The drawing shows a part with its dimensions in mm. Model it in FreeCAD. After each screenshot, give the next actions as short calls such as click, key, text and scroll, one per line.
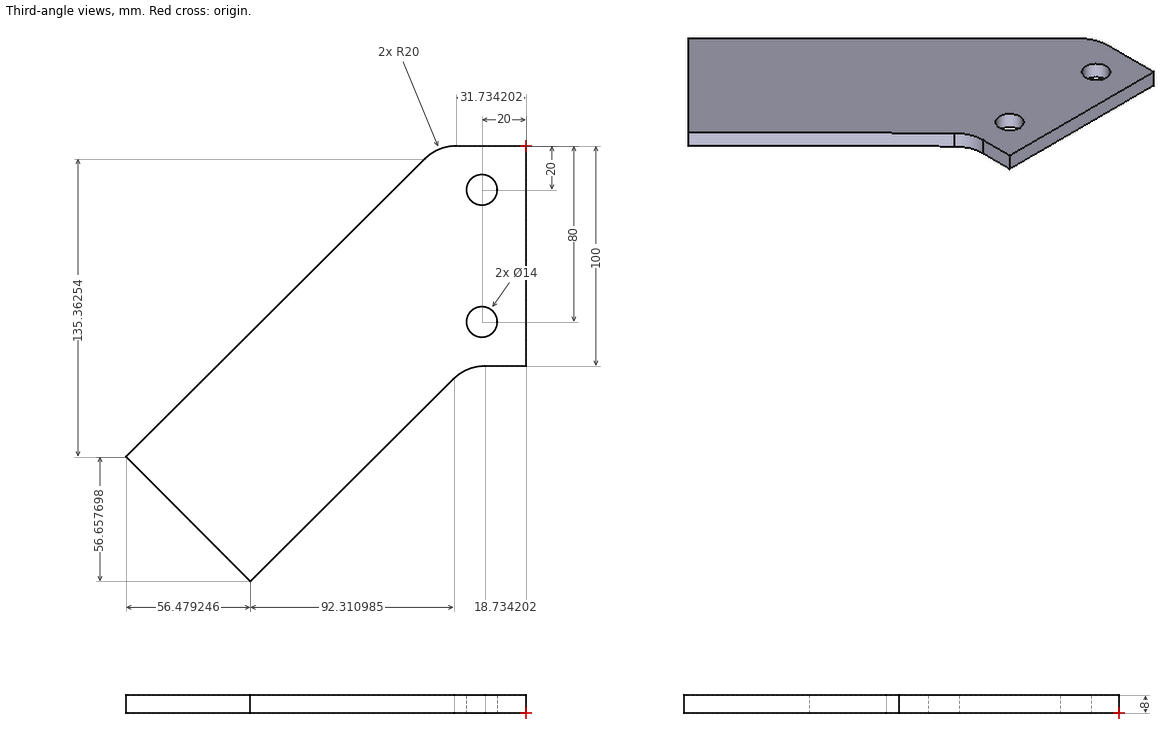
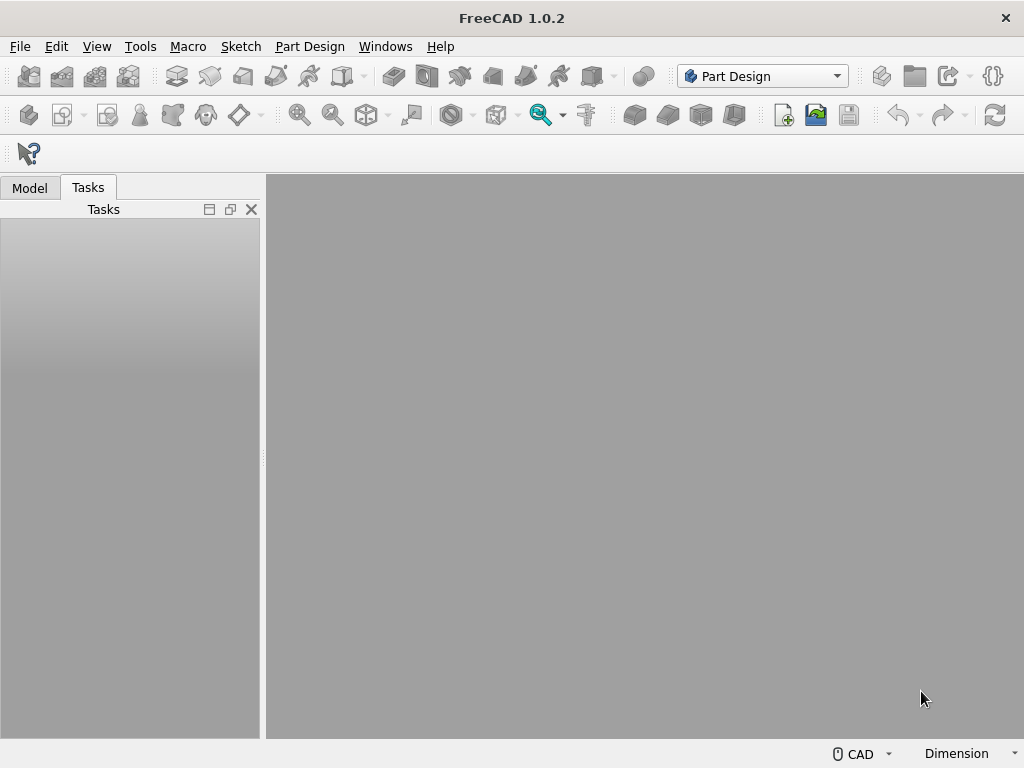
click(783, 116)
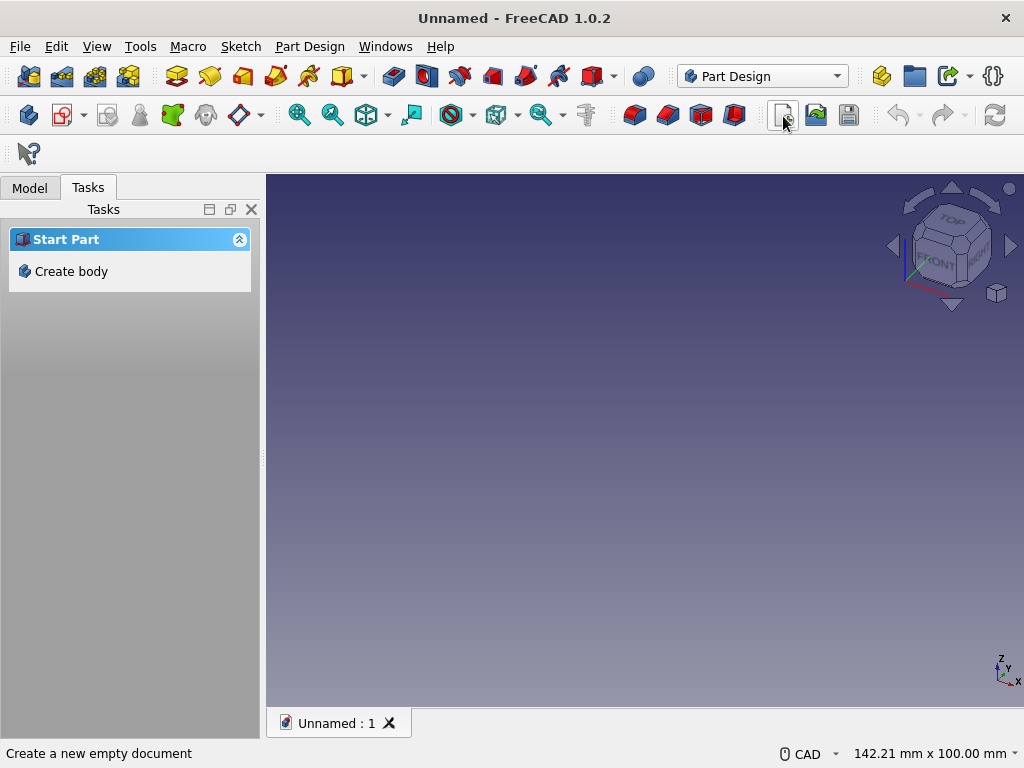
click(62, 116)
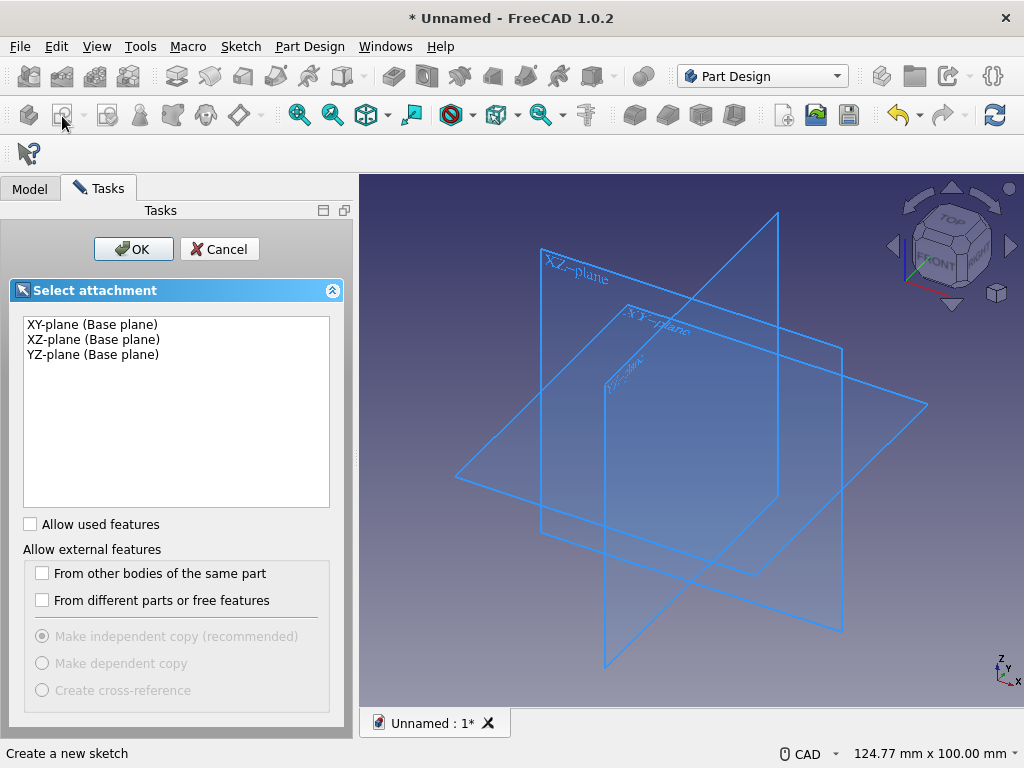
click(84, 324)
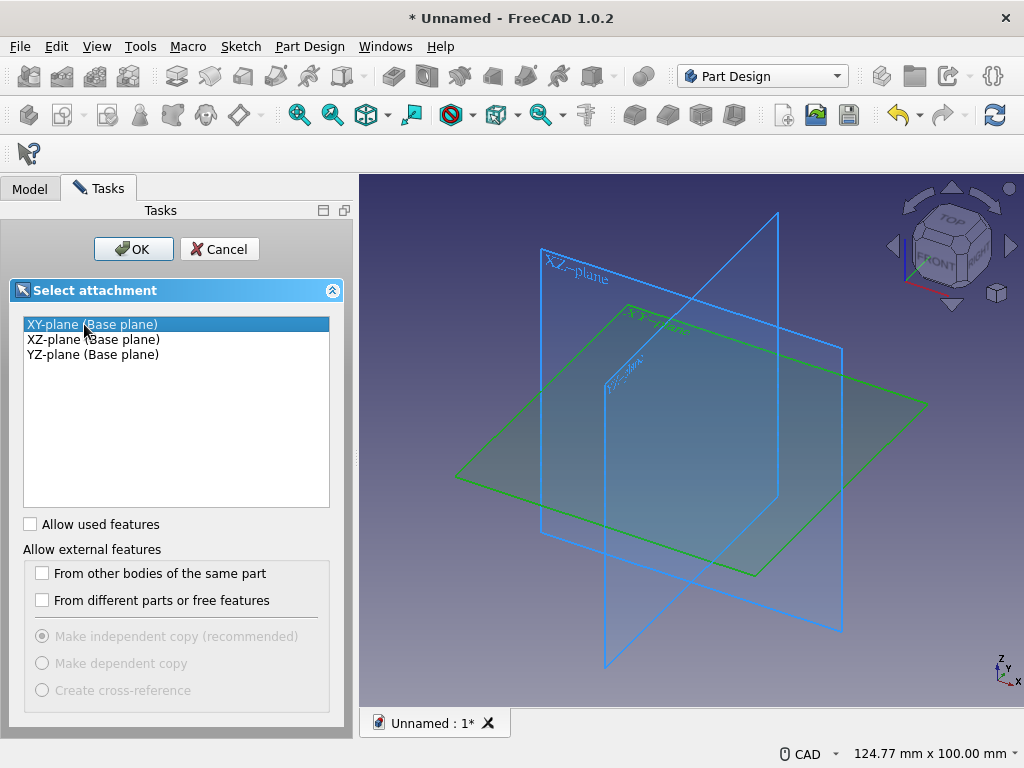
click(134, 249)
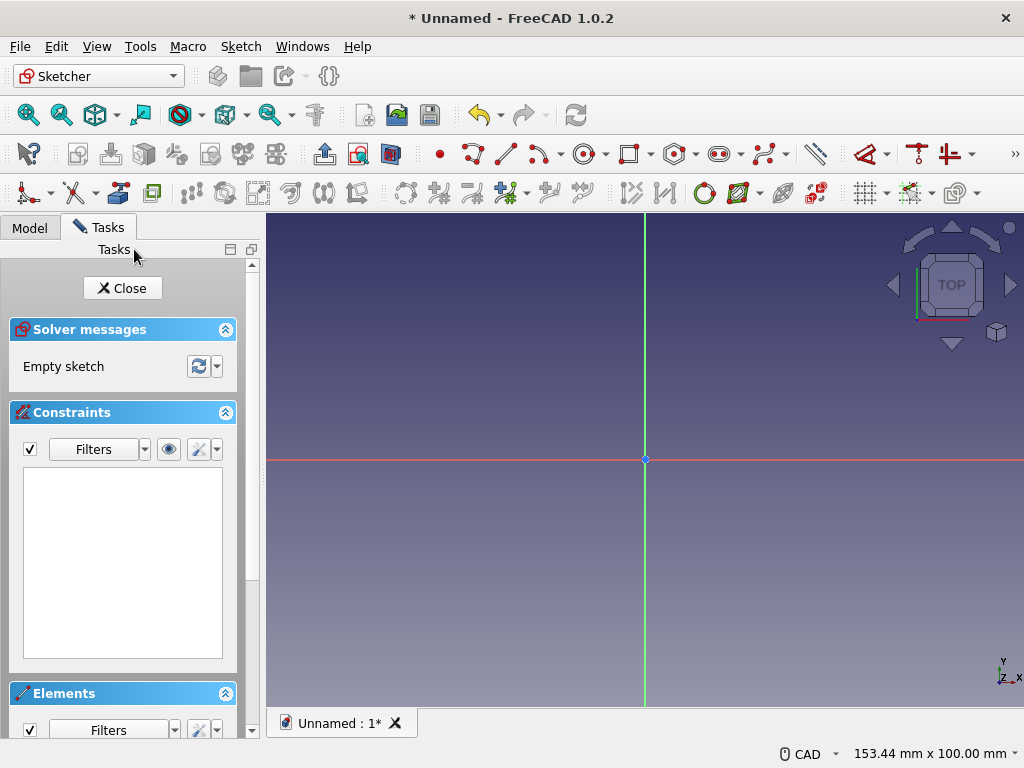
scroll(740, 249, down, 6)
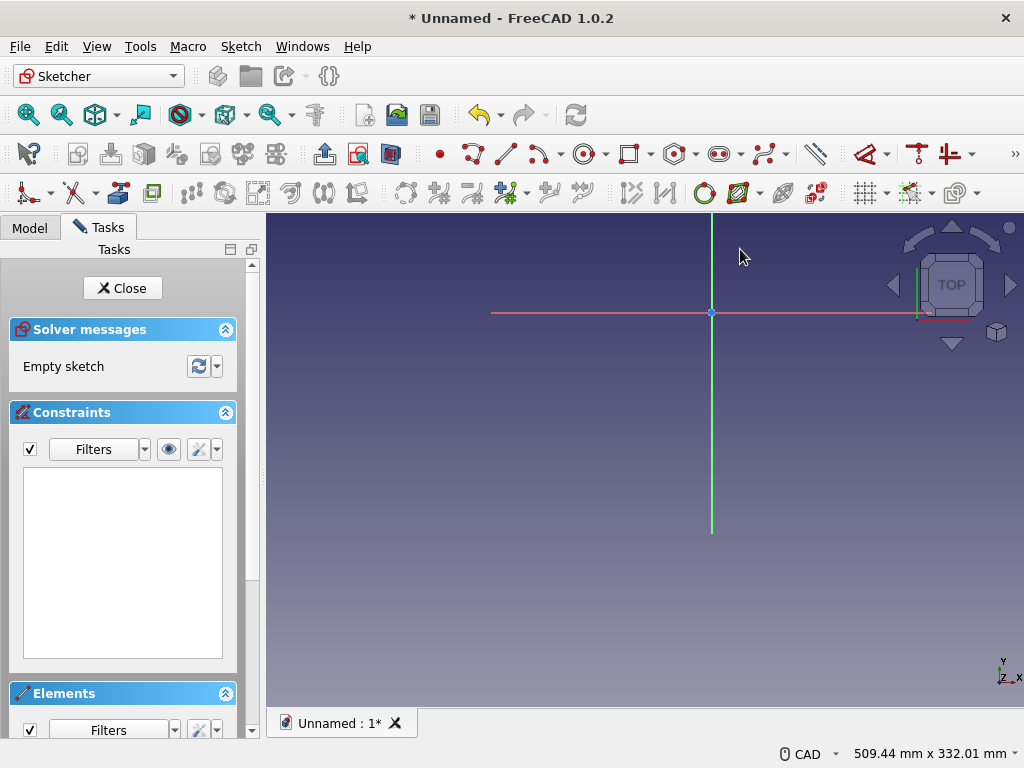
click(473, 154)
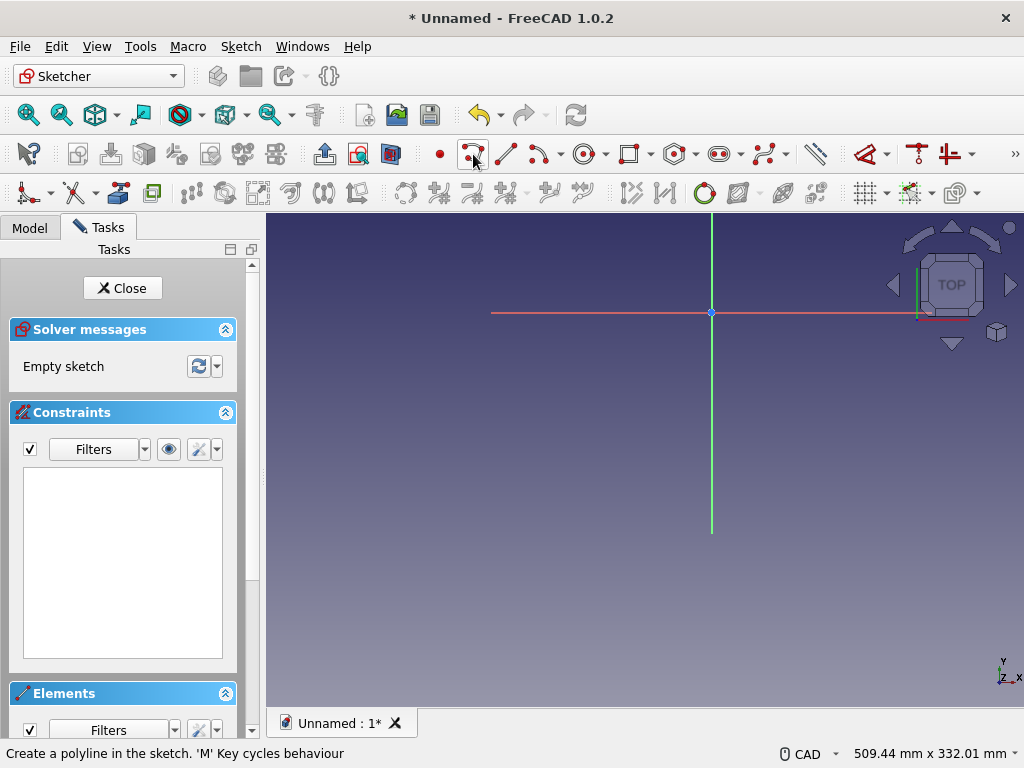
scroll(644, 321, up, 4)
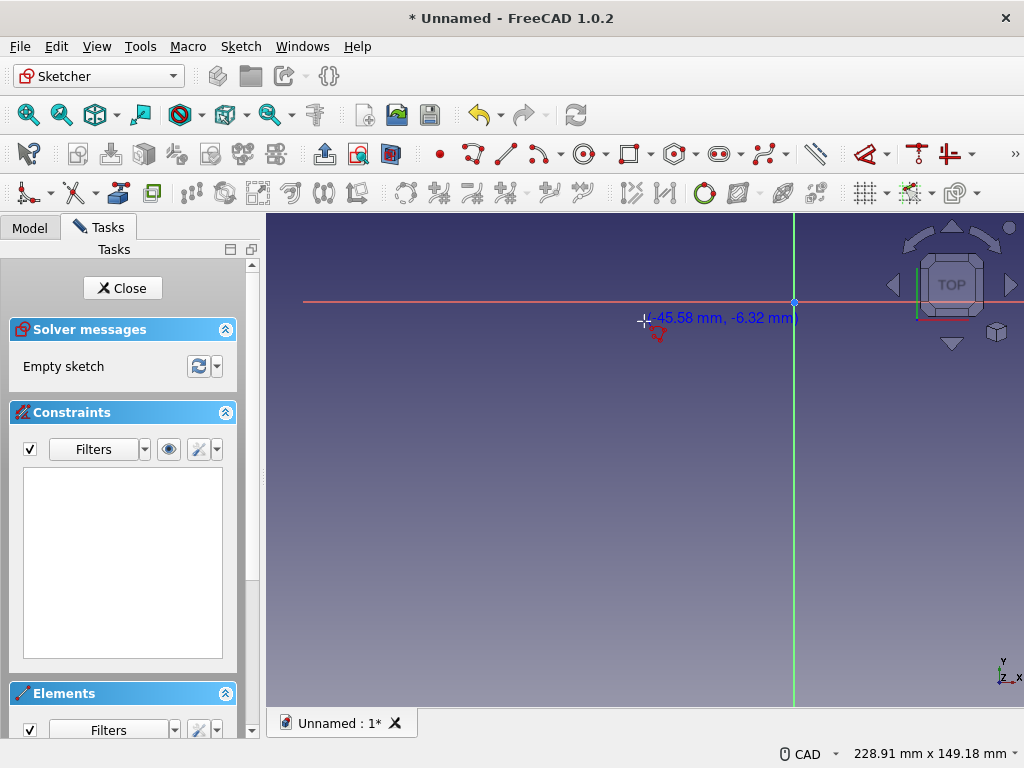
click(642, 321)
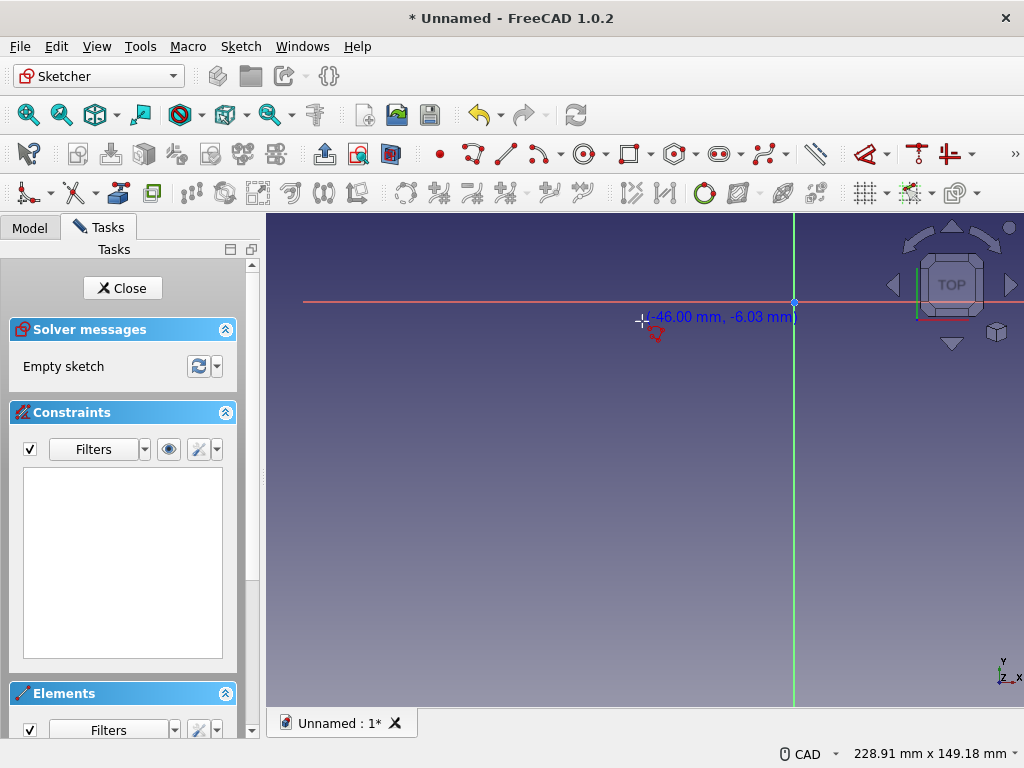
scroll(644, 322, down, 4)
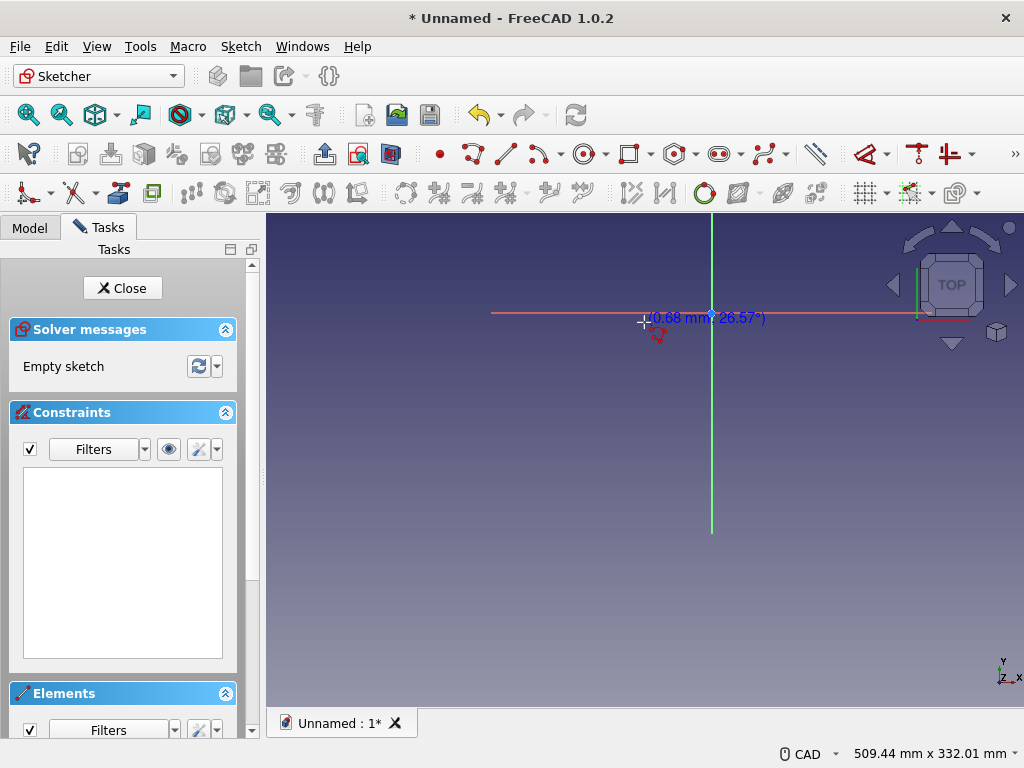
click(442, 523)
click(526, 608)
click(663, 471)
right_click(663, 471)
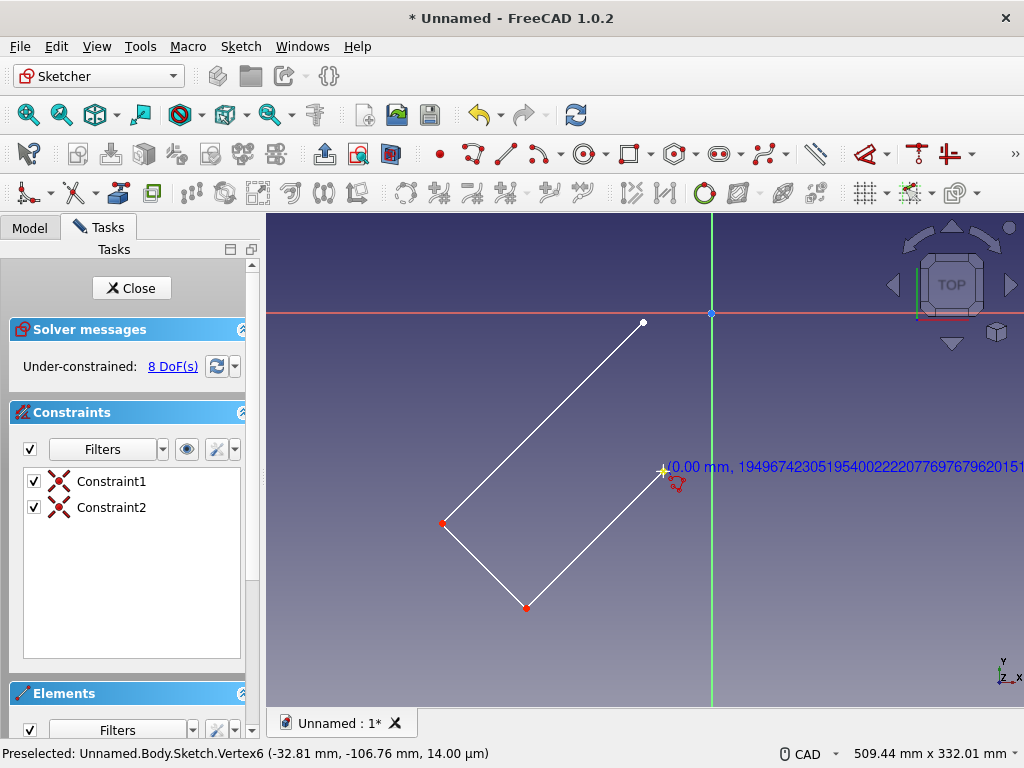
click(684, 462)
click(712, 462)
click(712, 313)
click(665, 322)
right_click(665, 322)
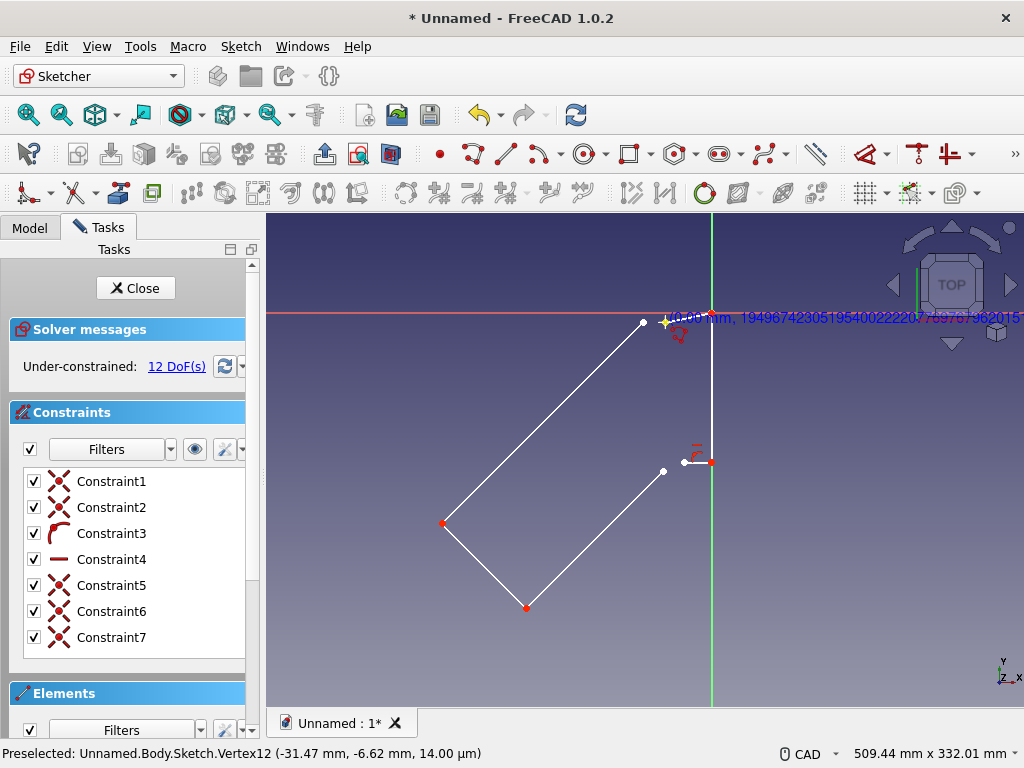
key(g)
key(3)
key(a)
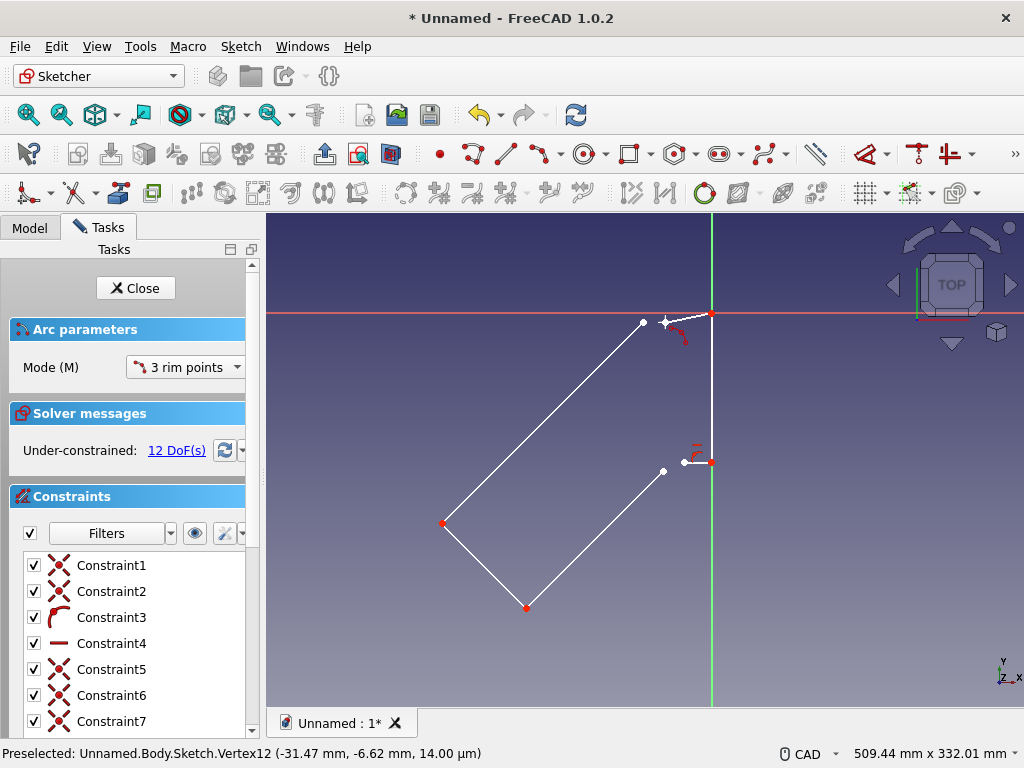
click(663, 472)
click(684, 463)